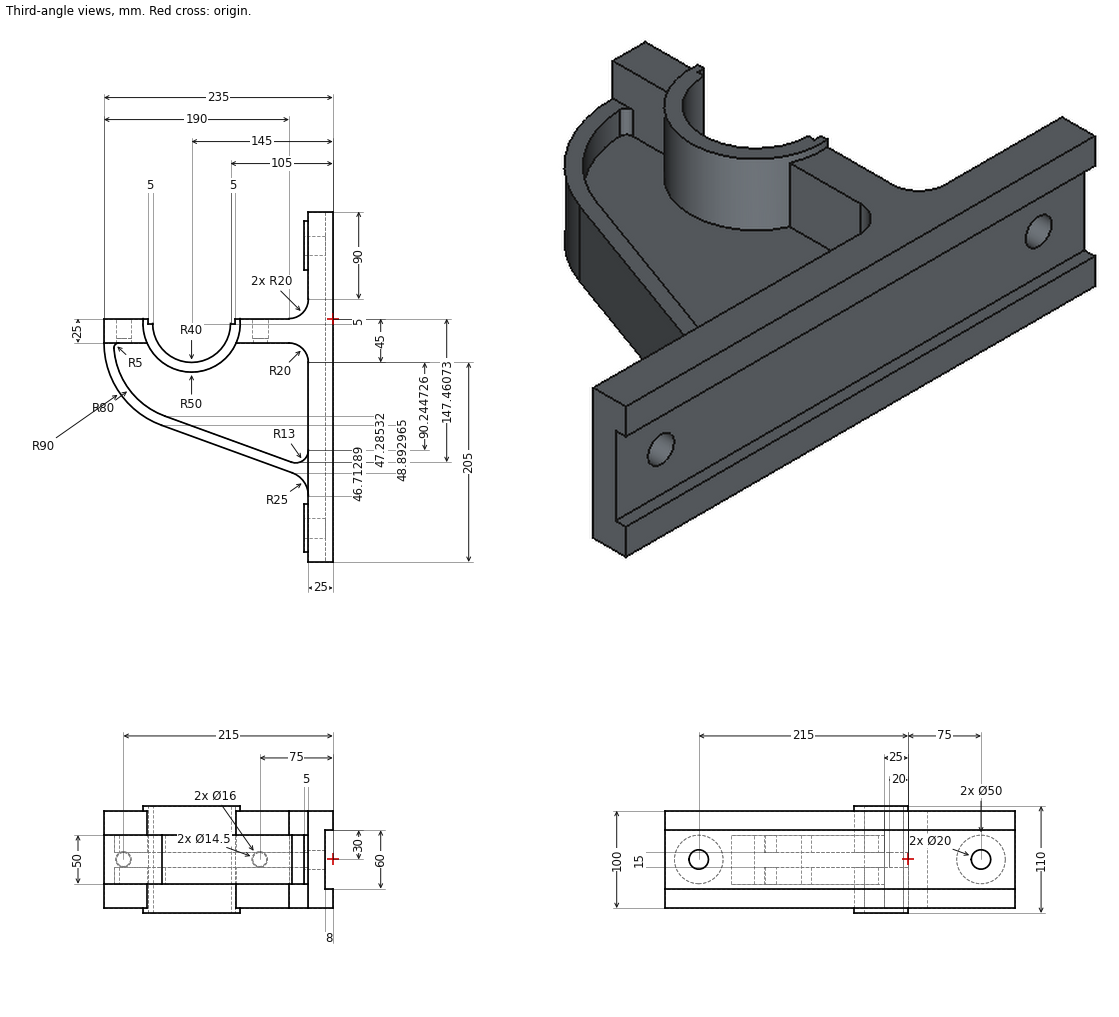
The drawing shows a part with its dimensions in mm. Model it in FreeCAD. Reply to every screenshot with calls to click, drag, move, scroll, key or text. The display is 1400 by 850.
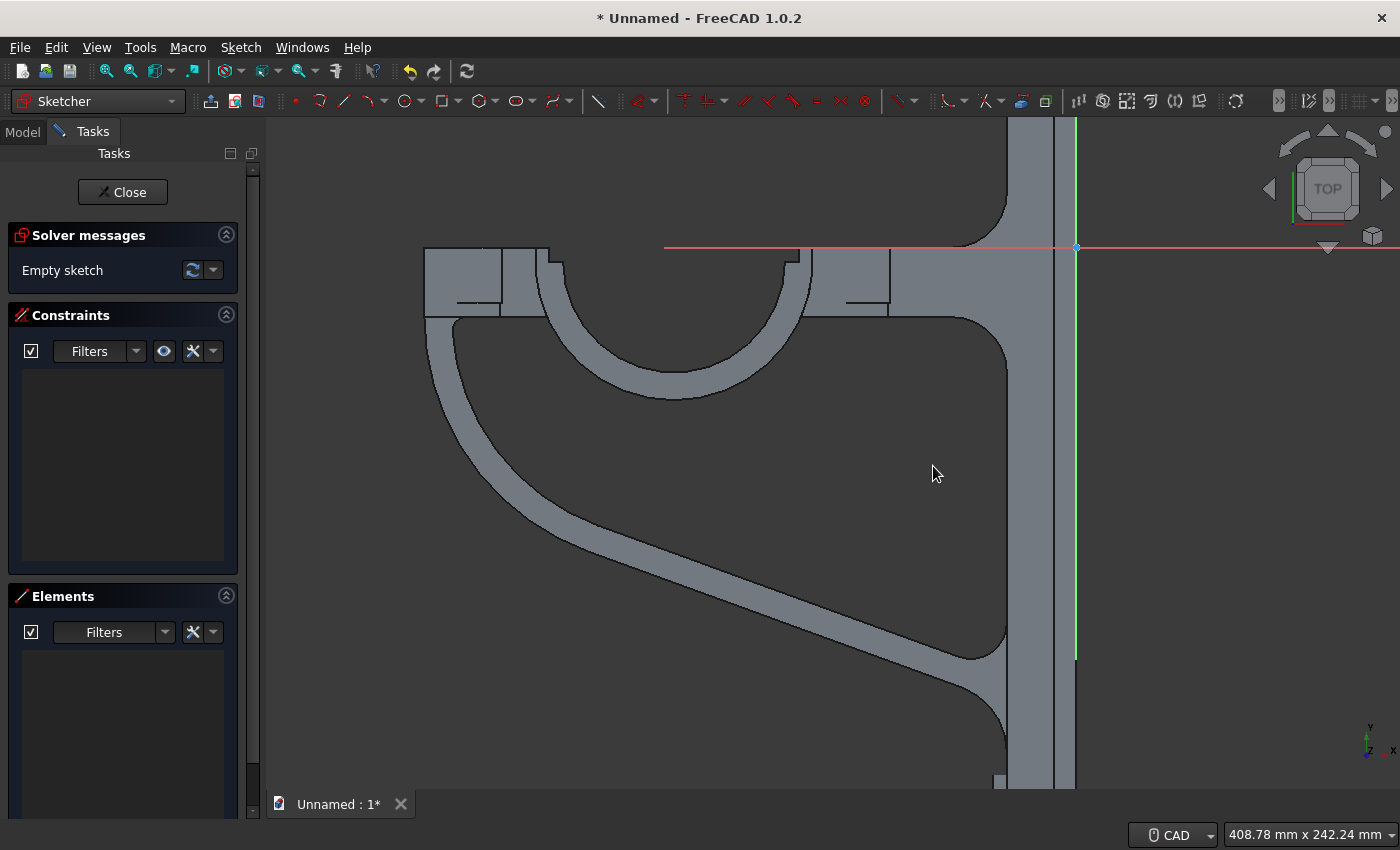
click(344, 102)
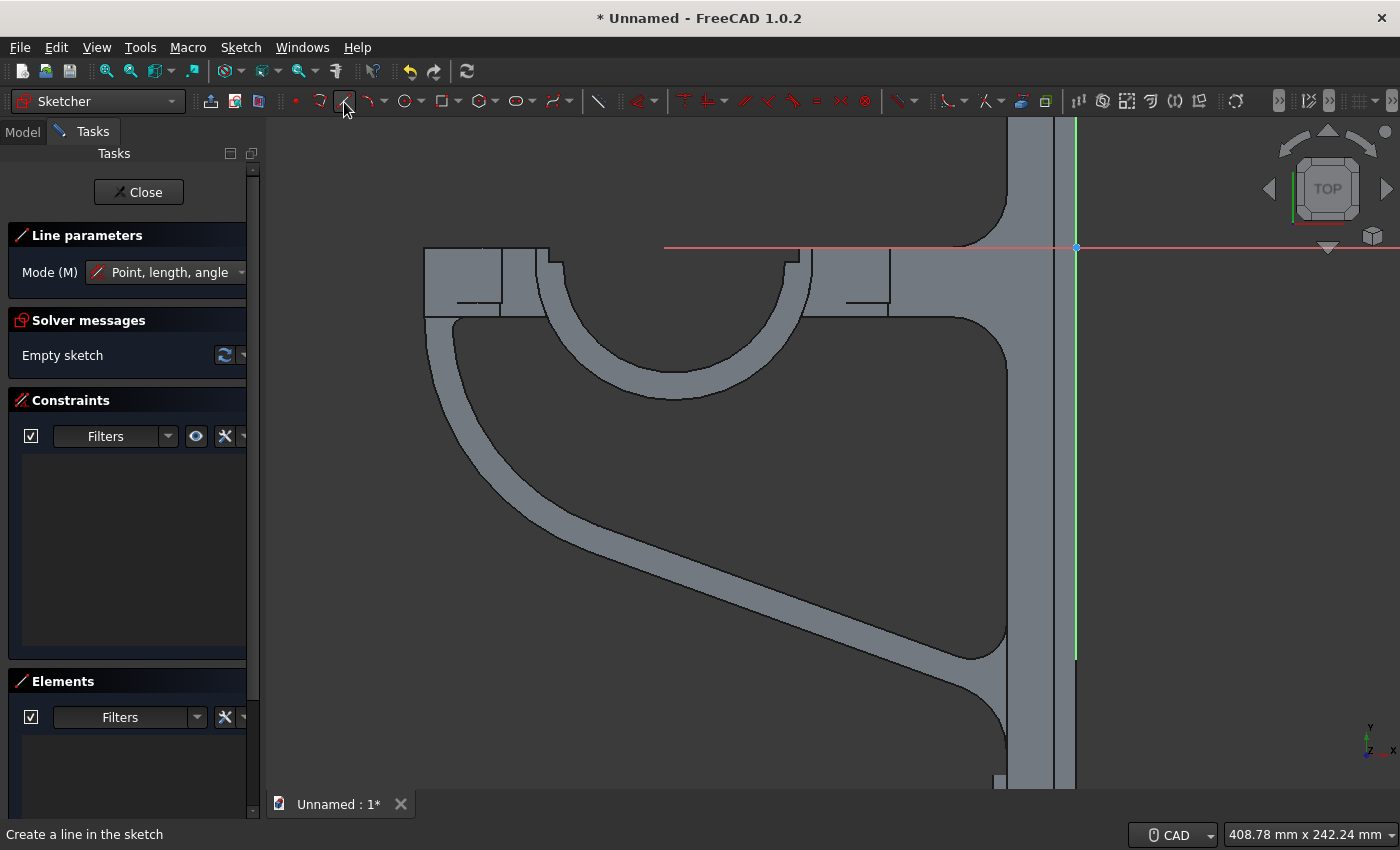
click(1007, 623)
click(1007, 373)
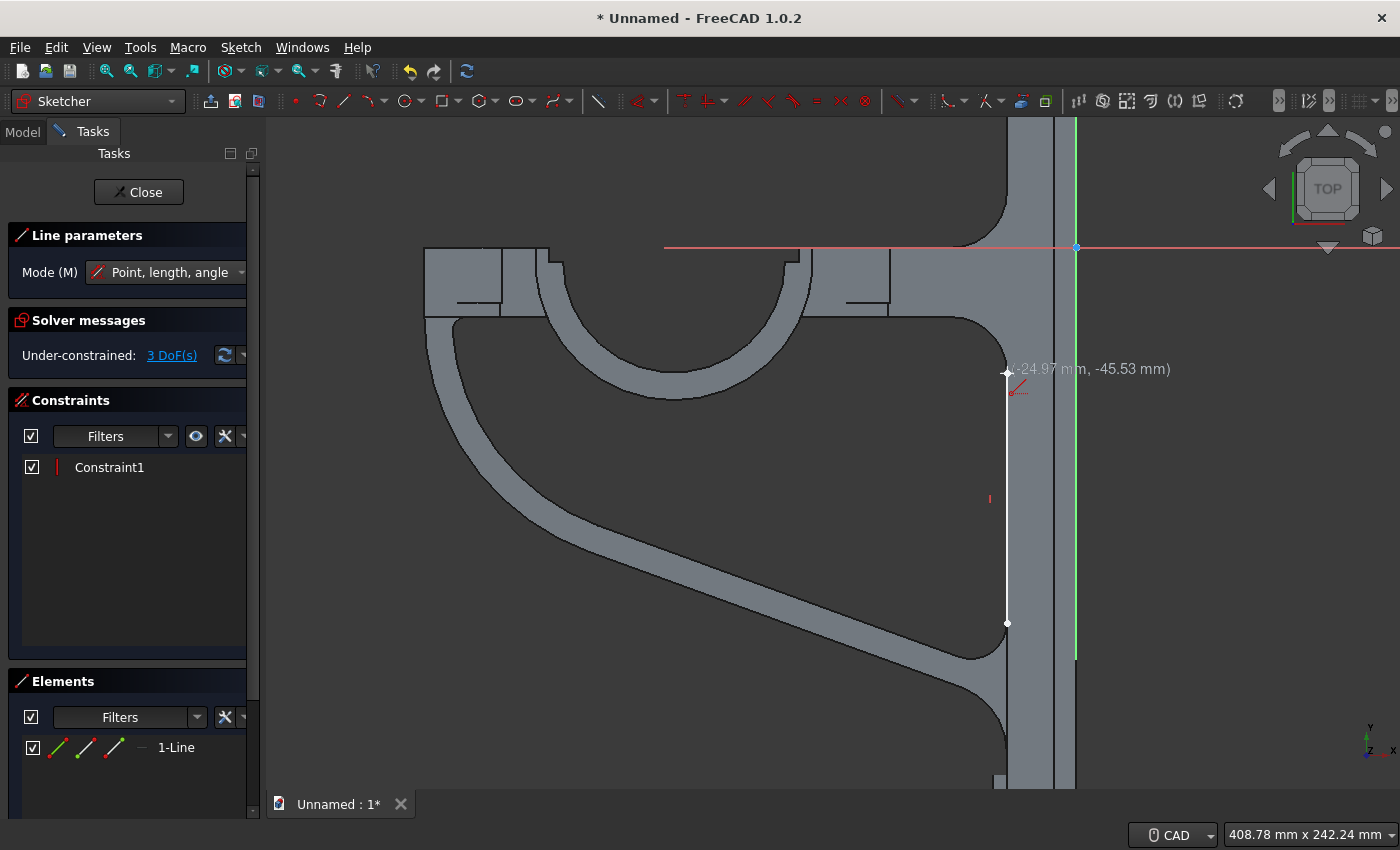
click(951, 317)
click(801, 317)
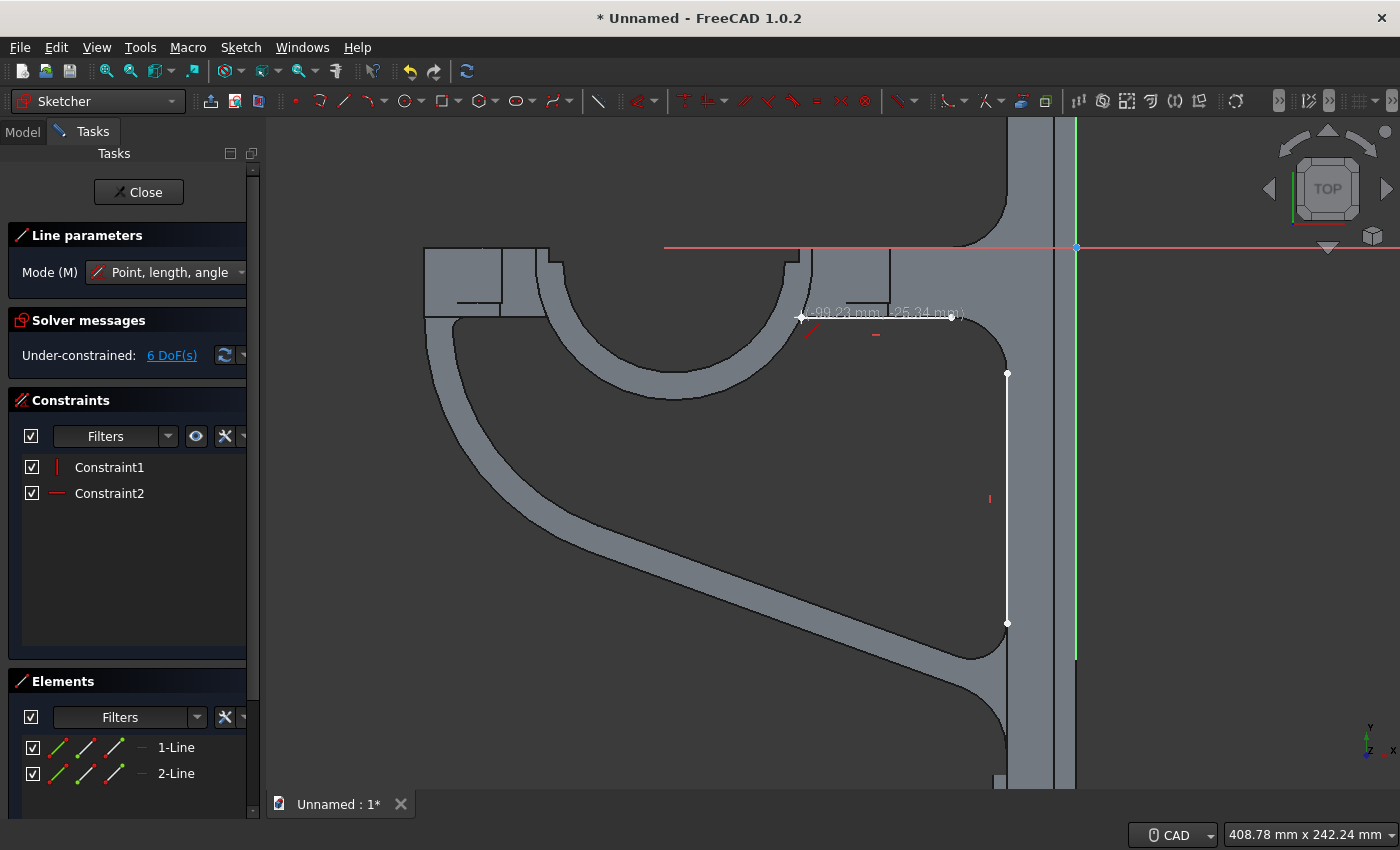
click(547, 317)
click(466, 317)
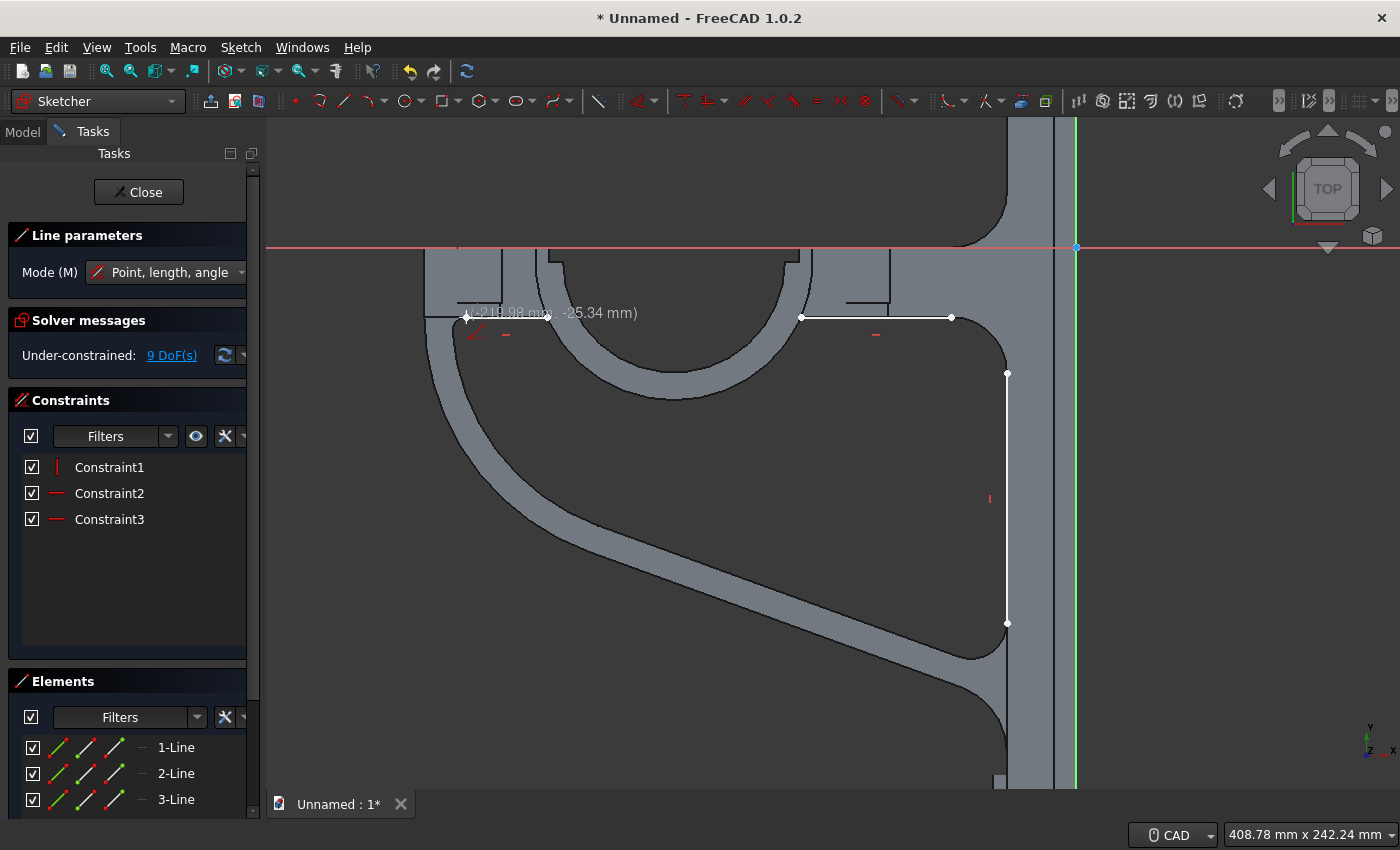
click(598, 526)
click(959, 657)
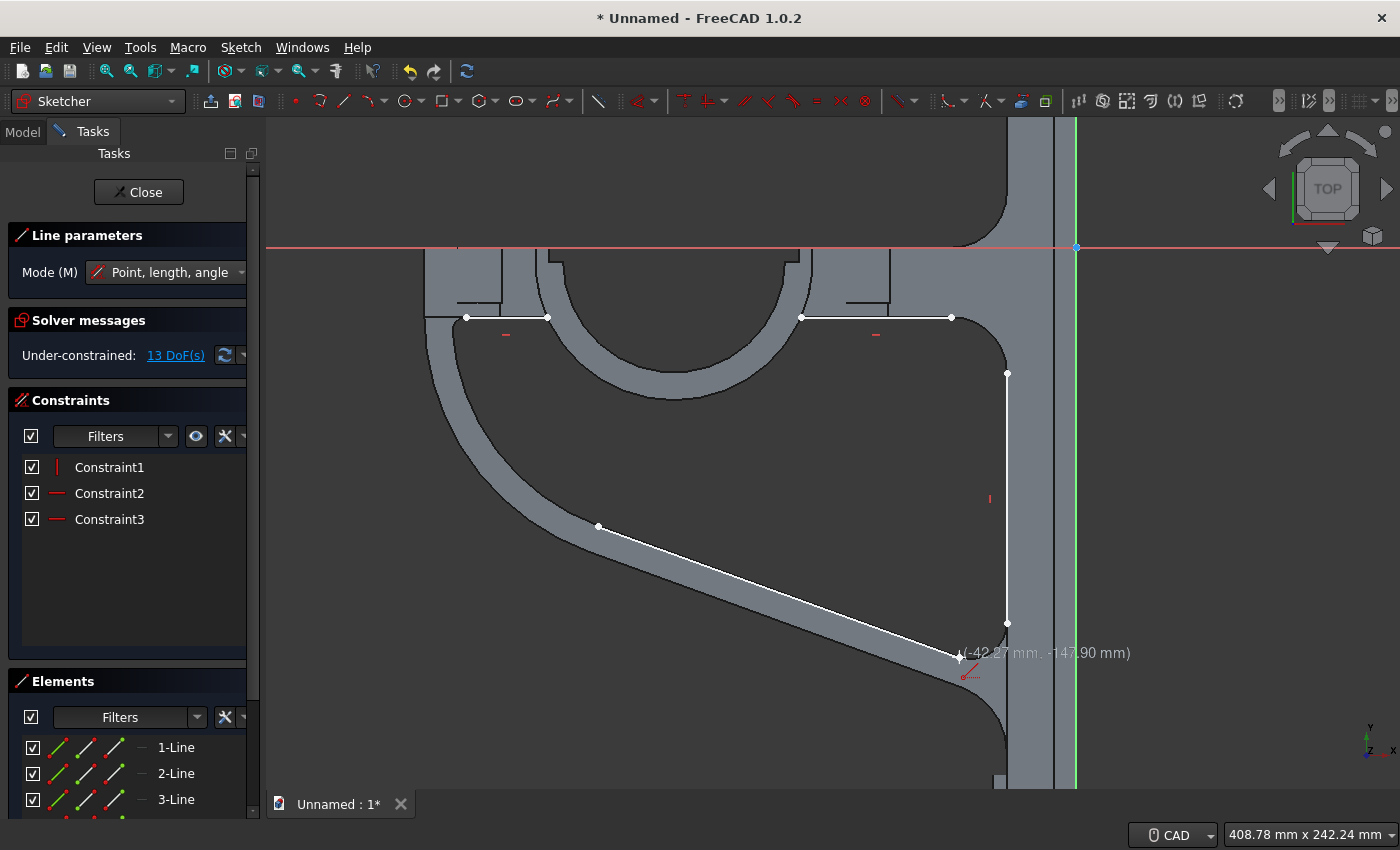
click(368, 102)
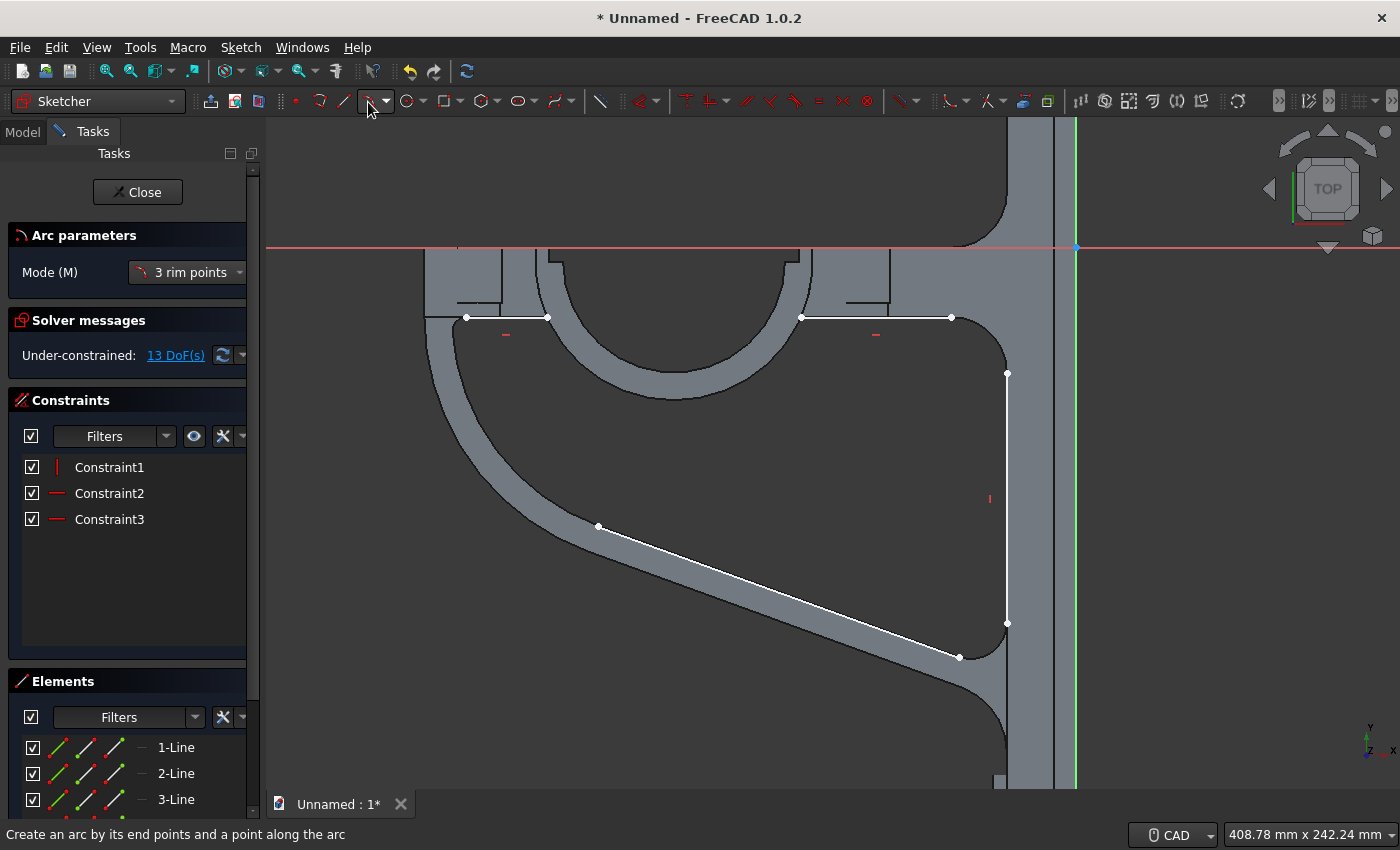
click(1007, 374)
click(951, 318)
click(991, 333)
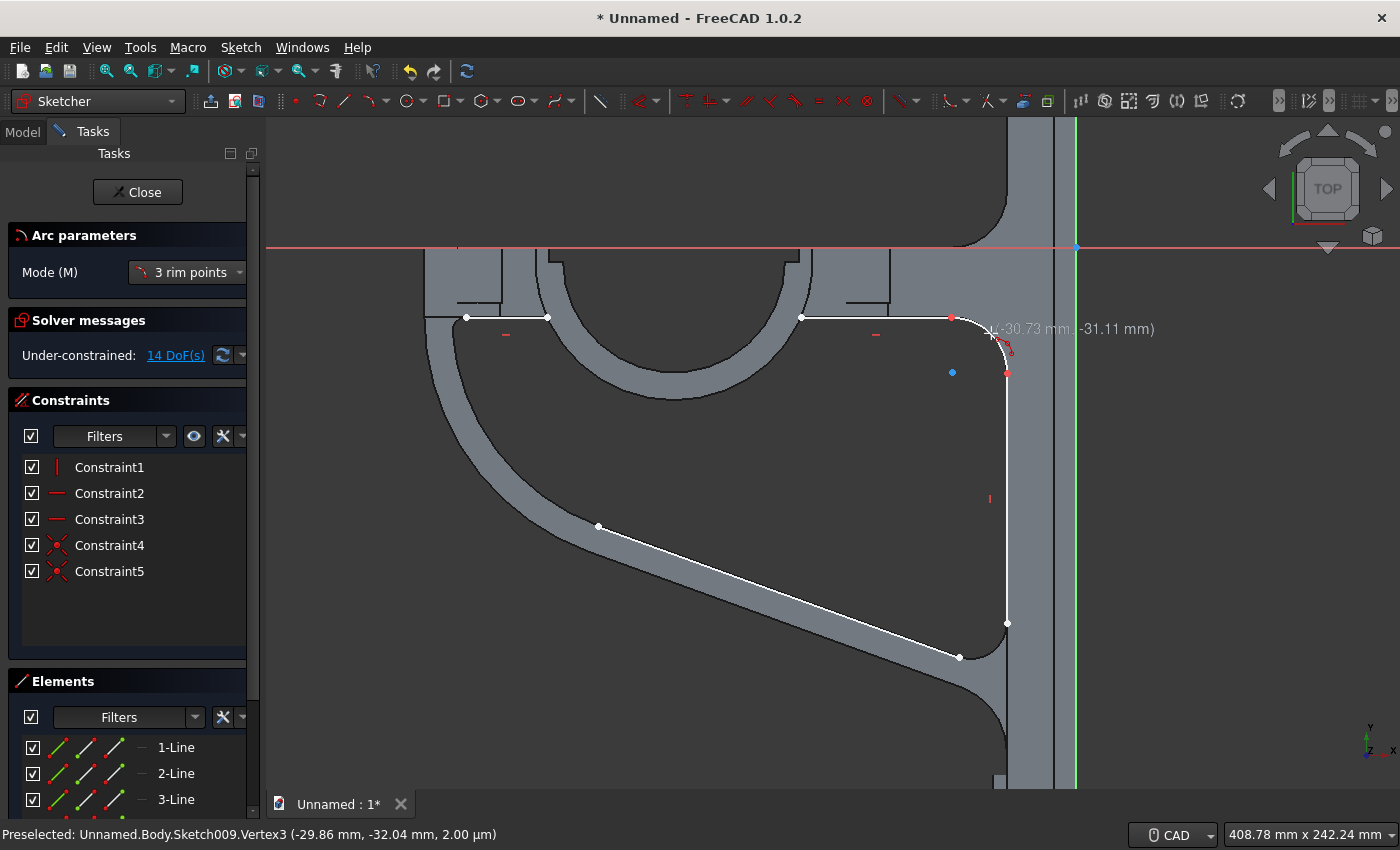
click(801, 318)
click(547, 318)
click(674, 400)